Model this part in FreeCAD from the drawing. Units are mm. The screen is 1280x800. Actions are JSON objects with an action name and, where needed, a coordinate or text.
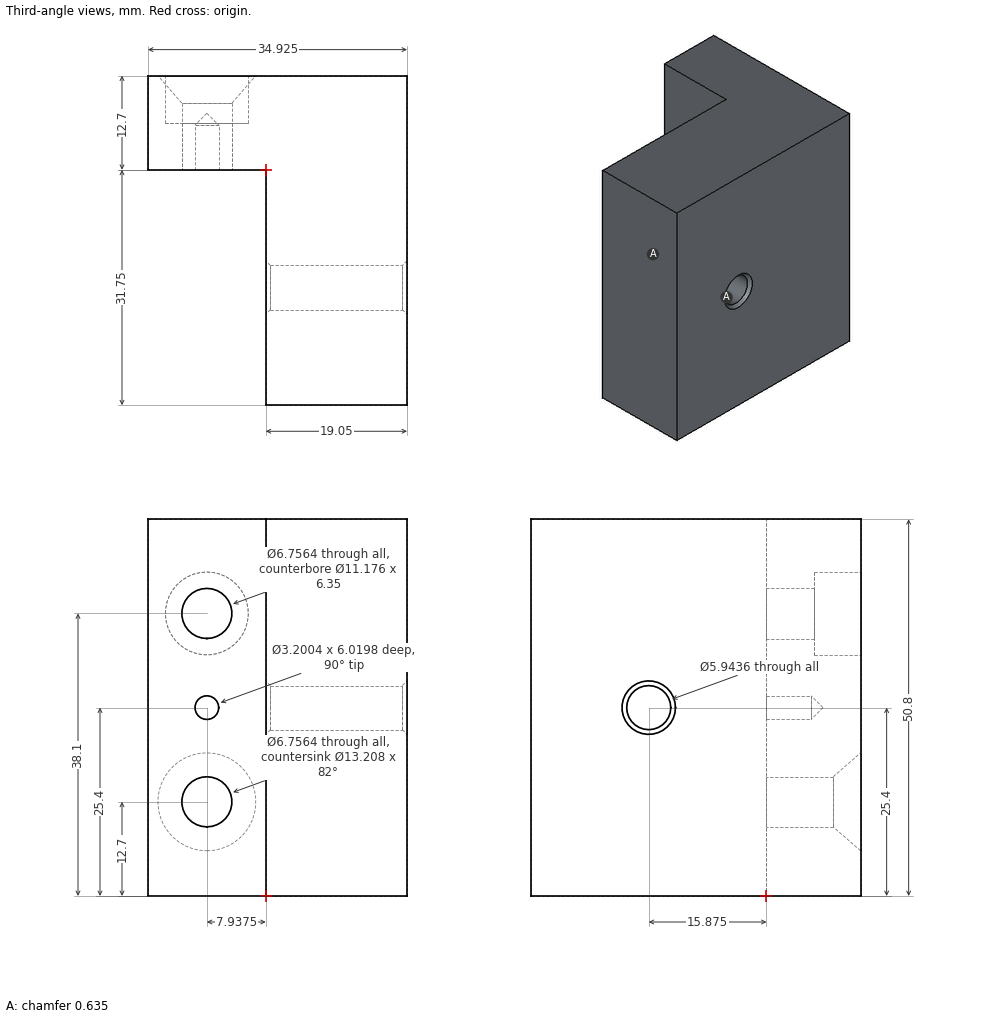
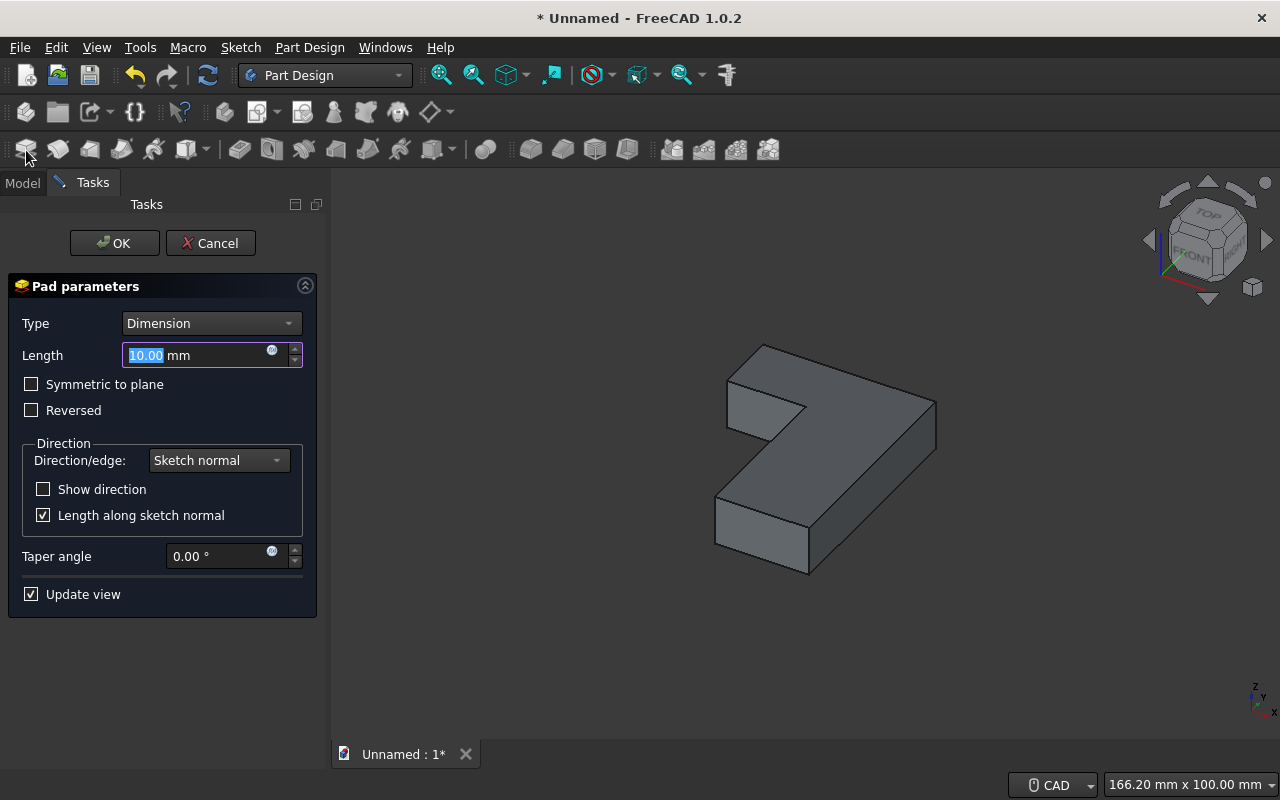
{"action": "type", "text": "50.8"}
{"action": "key", "text": "Tab"}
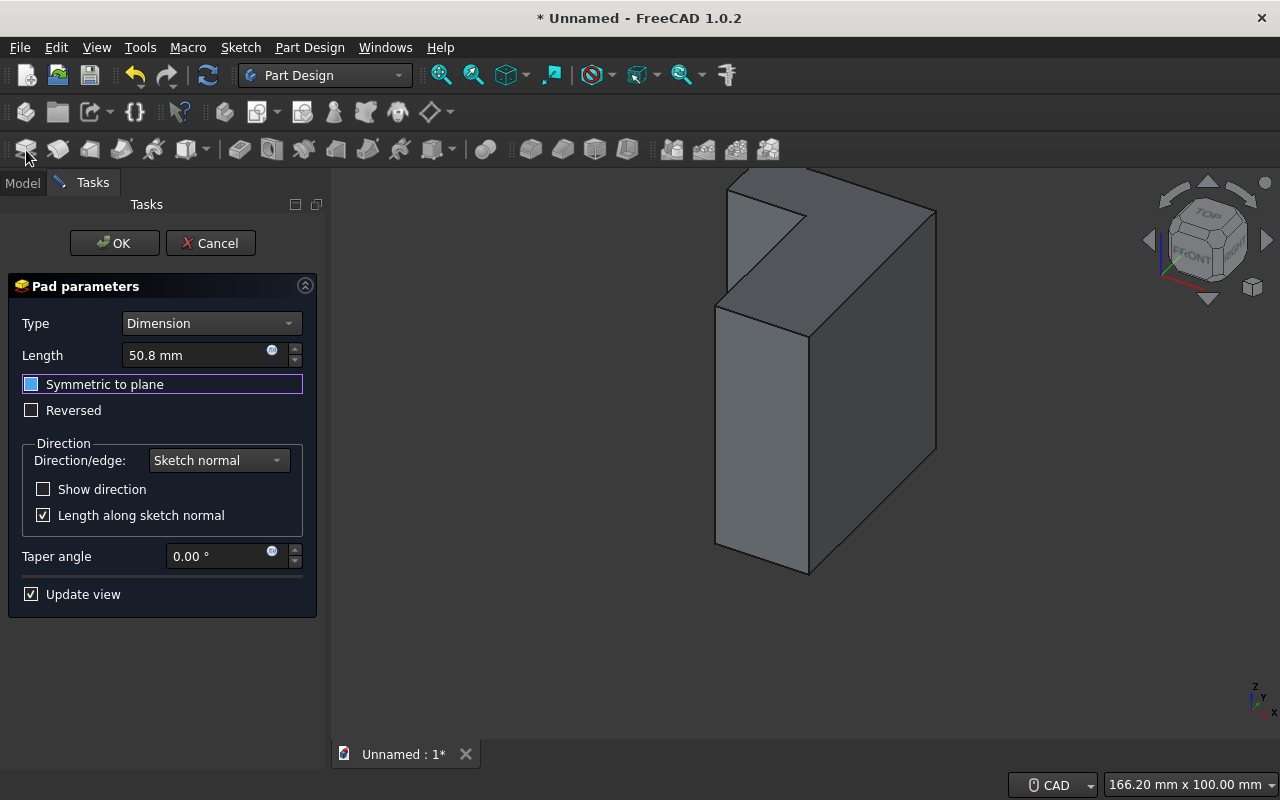
{"action": "left_click", "coordinate": [115, 243]}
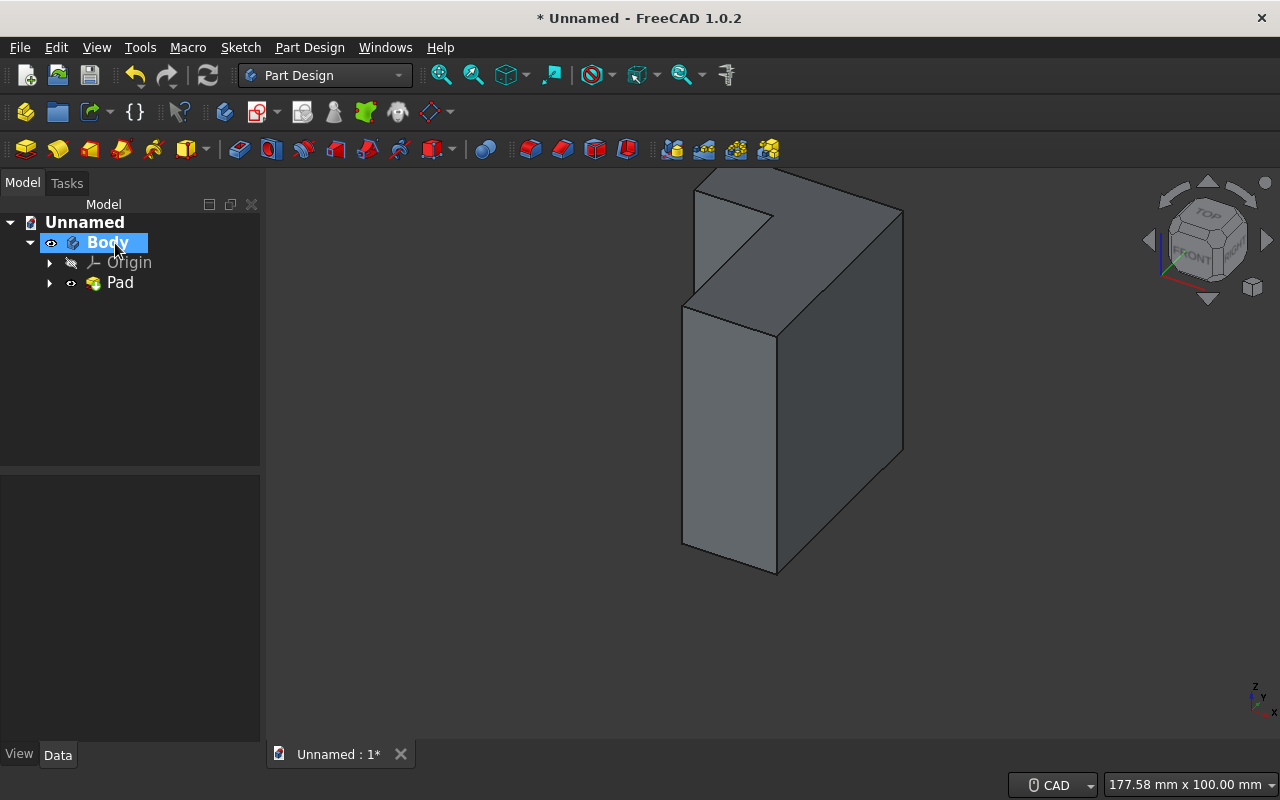
{"action": "left_click", "coordinate": [442, 76]}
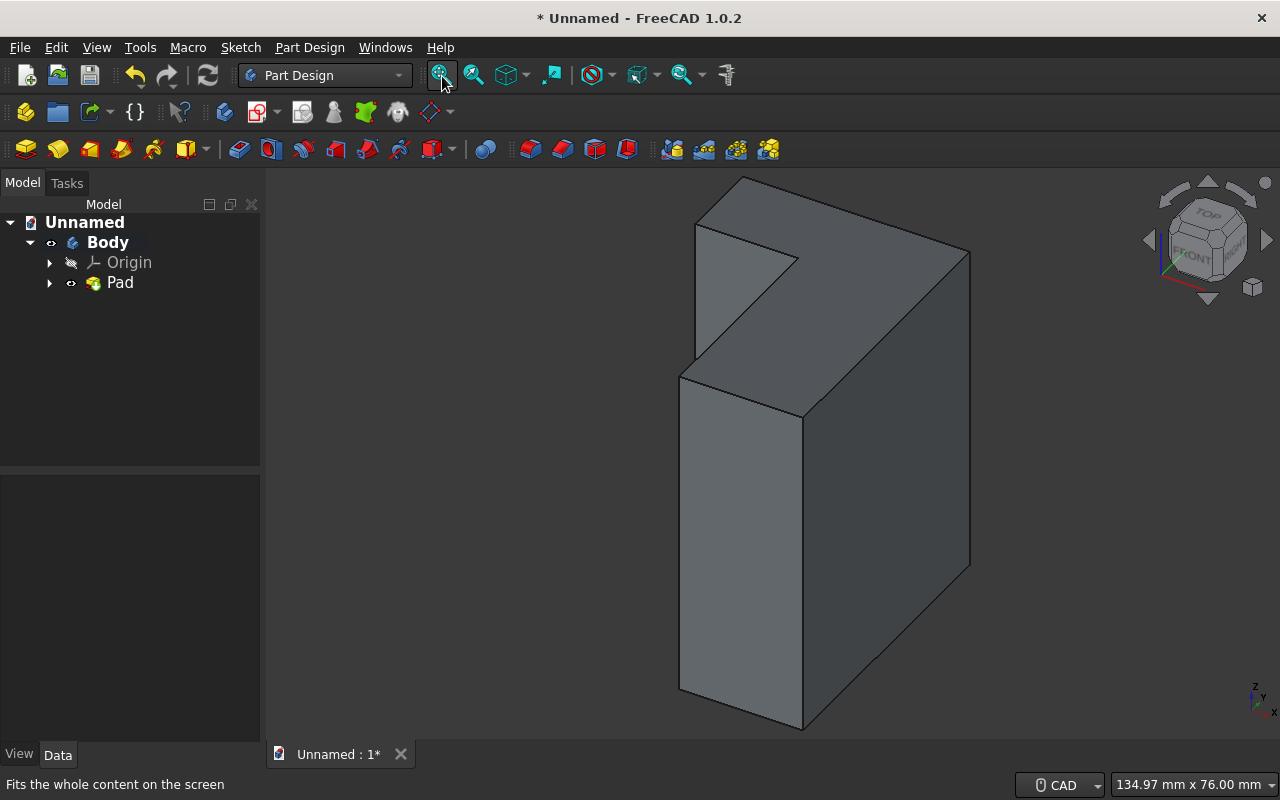
{"action": "key", "text": "6"}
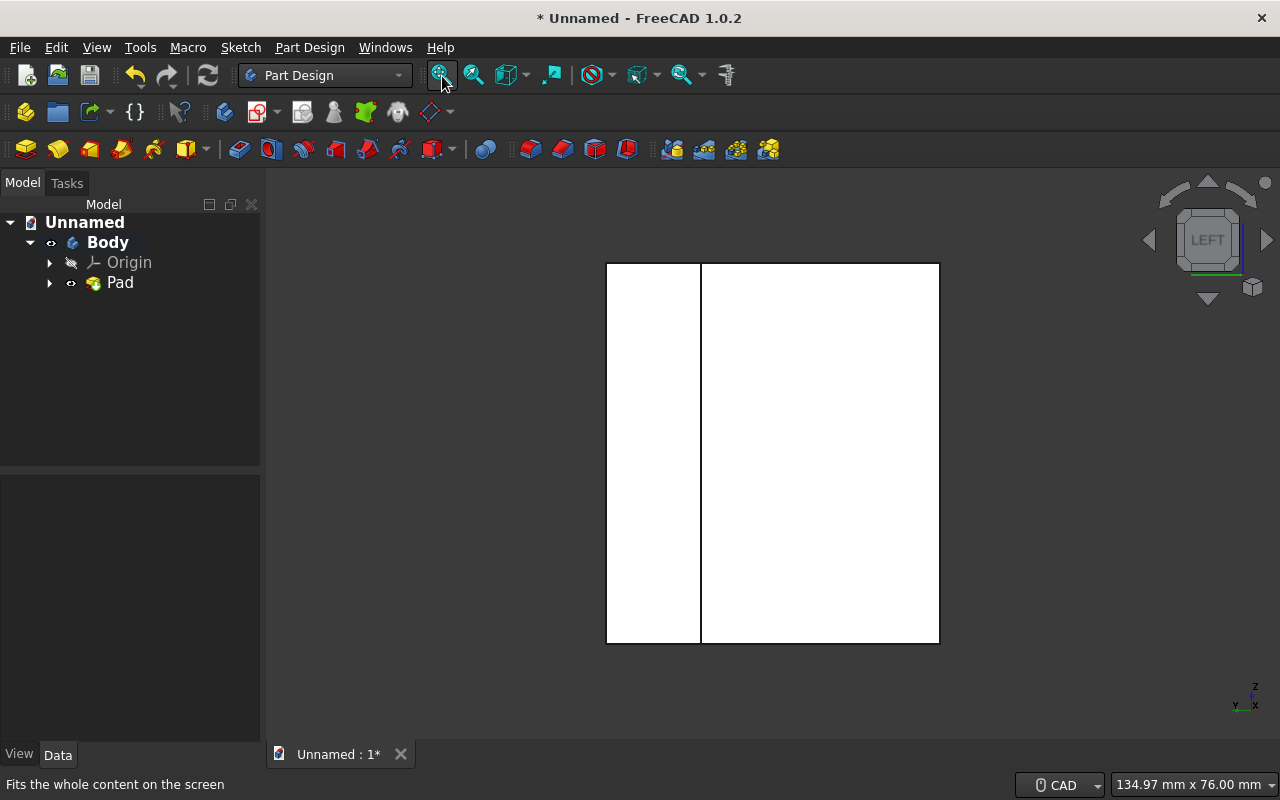
{"action": "left_click", "coordinate": [821, 398]}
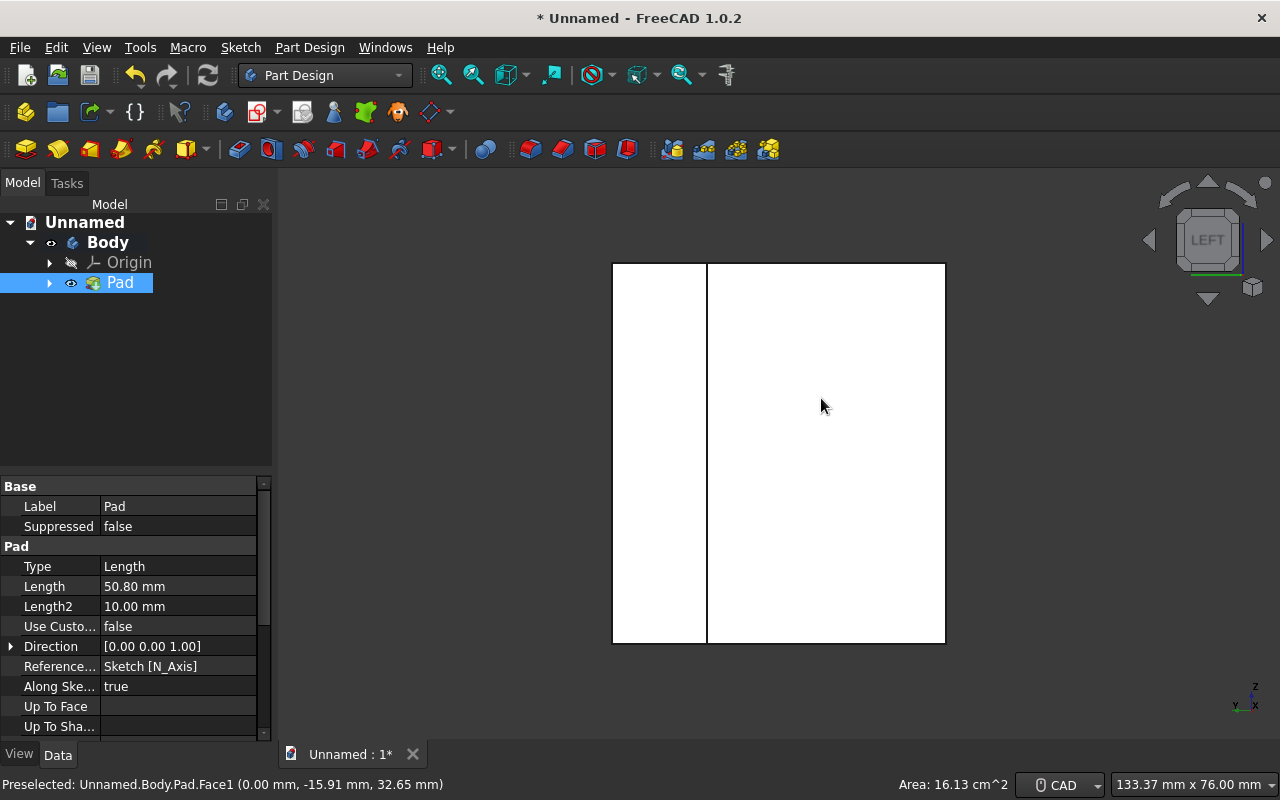
{"action": "left_click", "coordinate": [258, 112]}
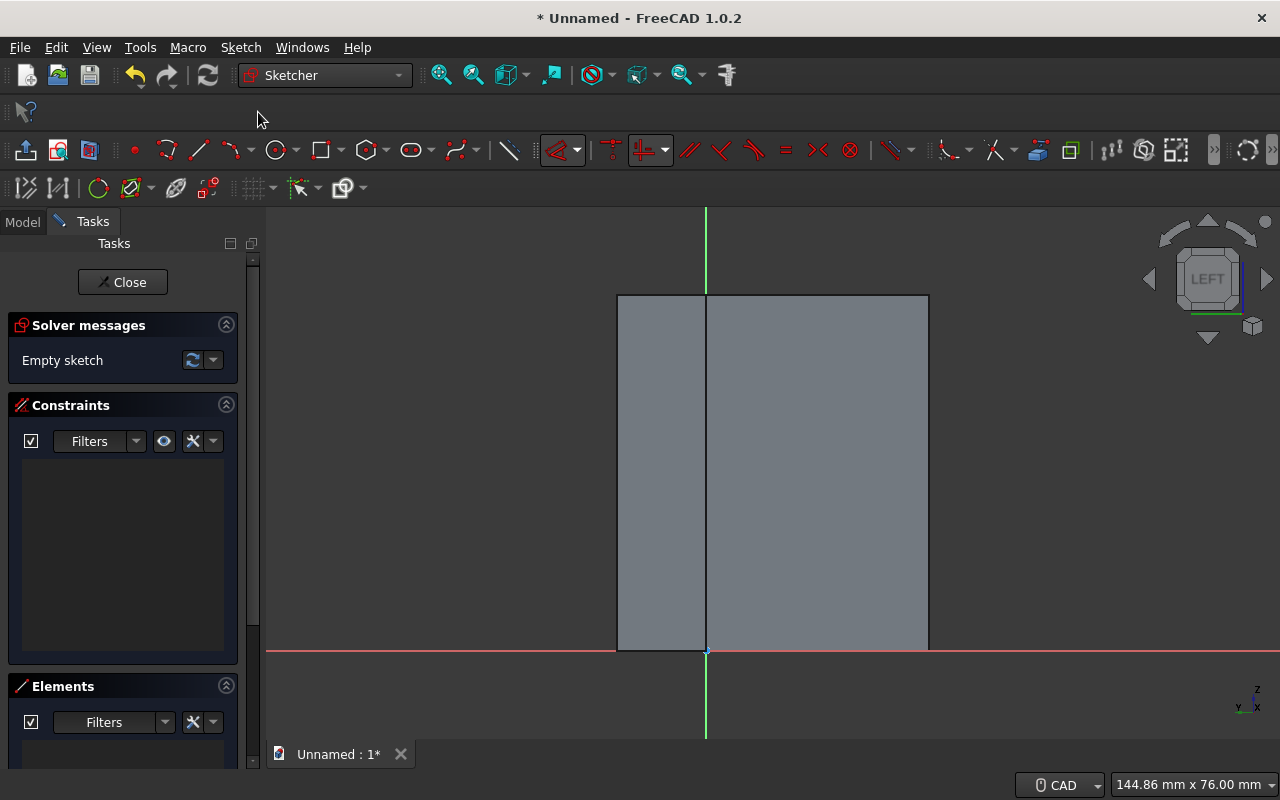
{"action": "left_click", "coordinate": [90, 150]}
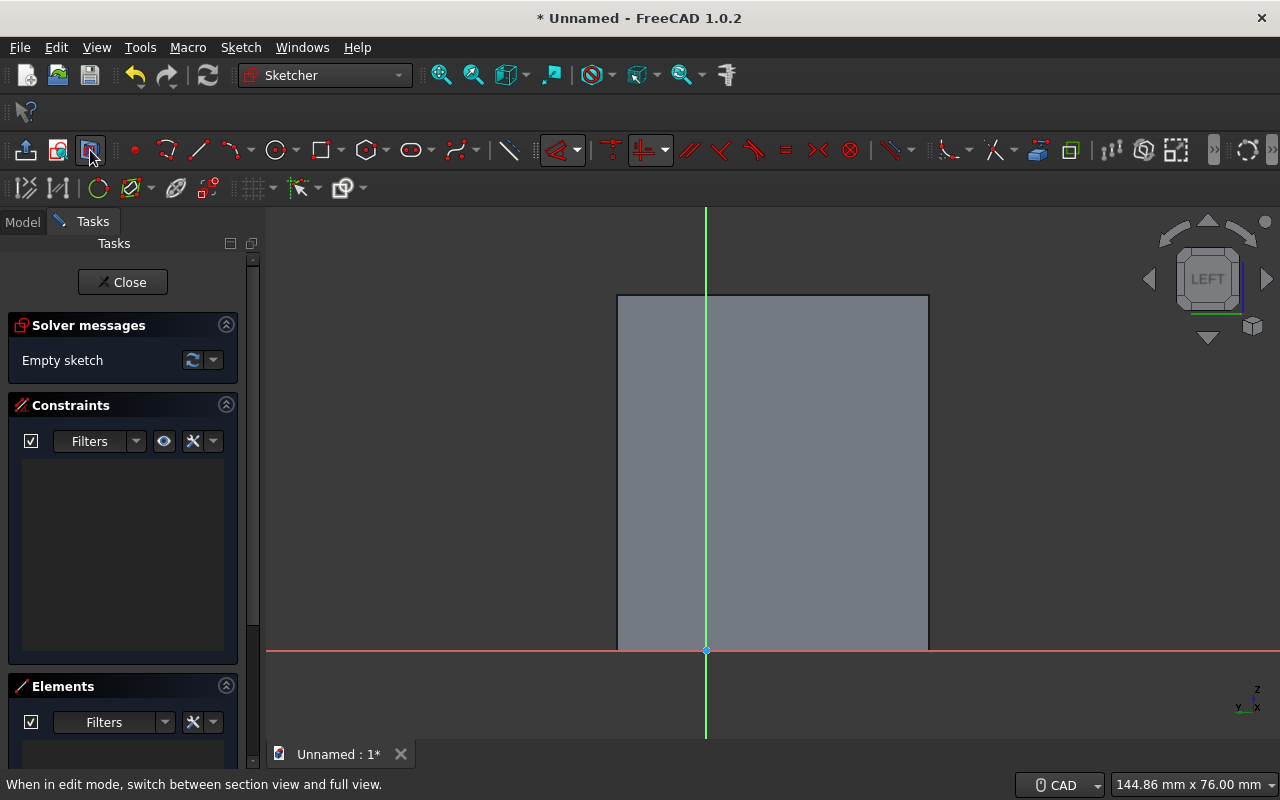
{"action": "scroll", "coordinate": [835, 473], "scroll_direction": "up", "scroll_amount": 10}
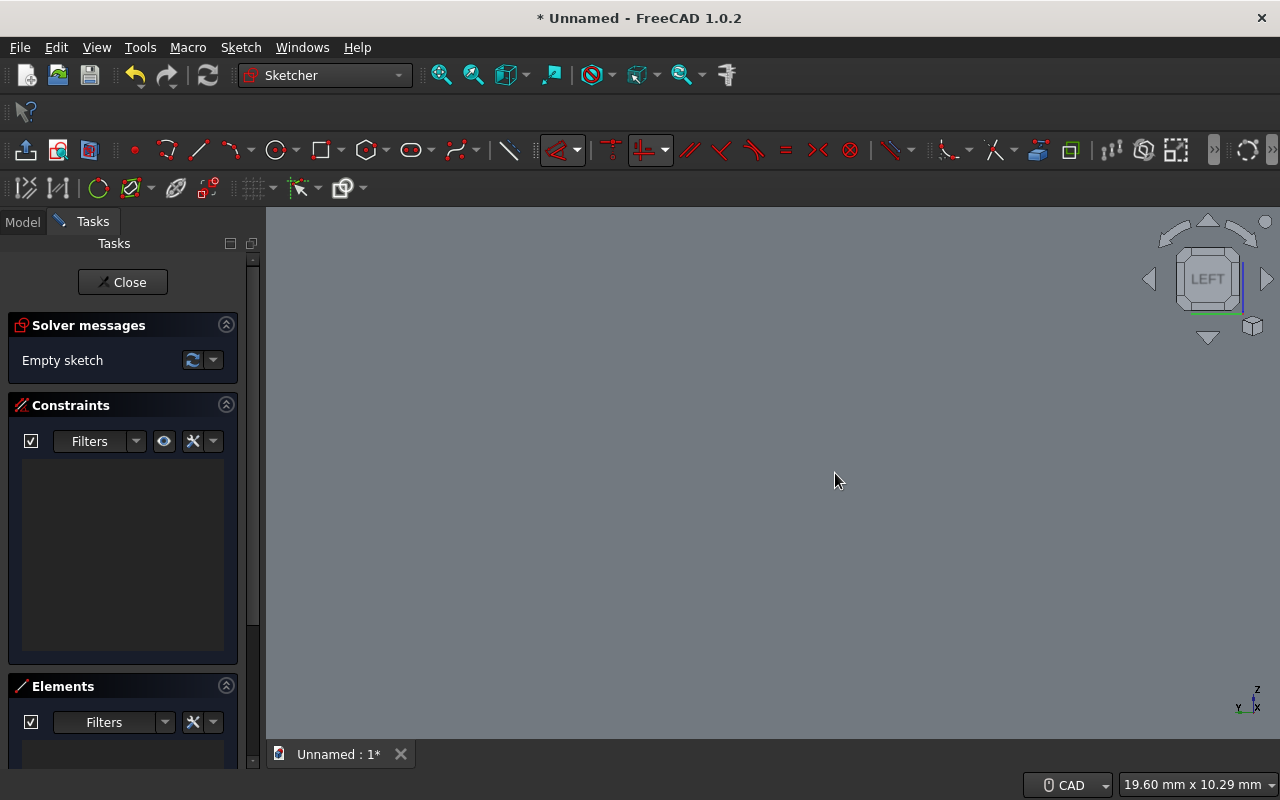
{"action": "left_click", "coordinate": [276, 150]}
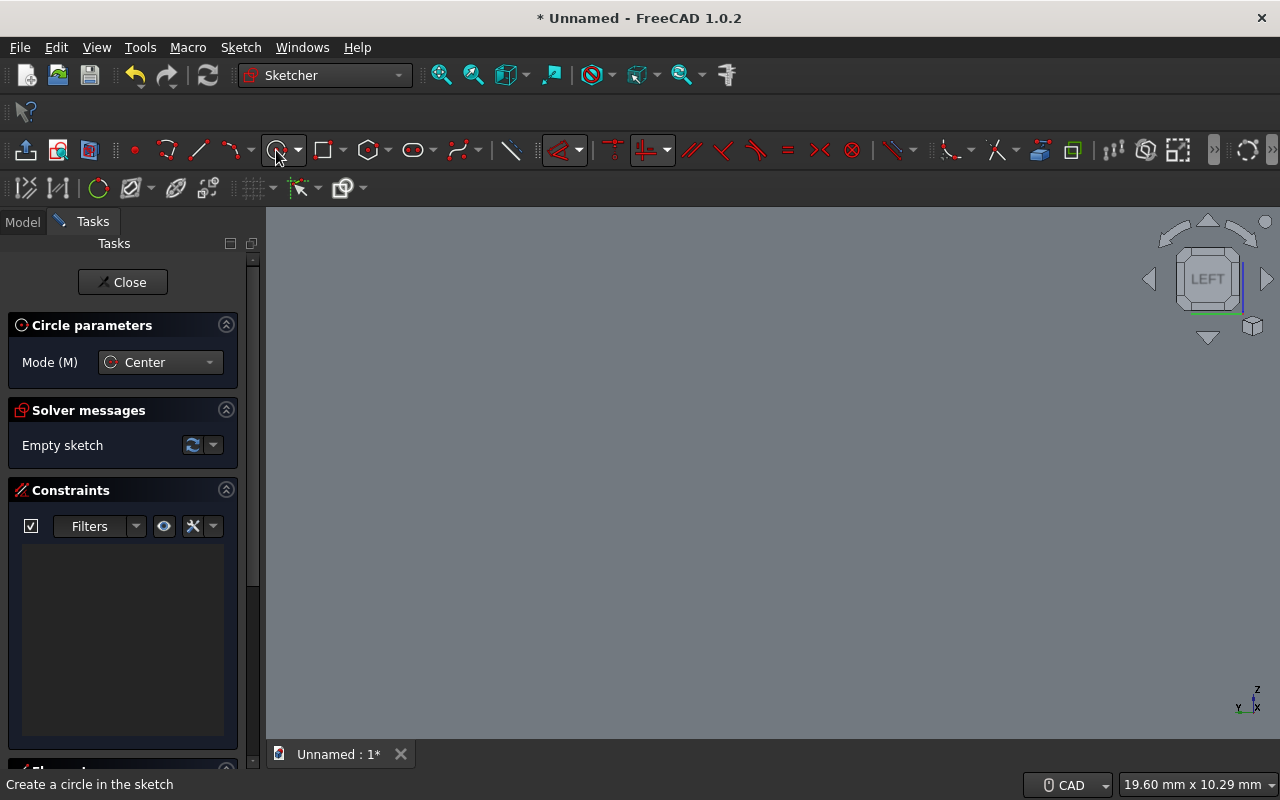
{"action": "left_click", "coordinate": [702, 470]}
{"action": "mouse_move", "coordinate": [810, 361]}